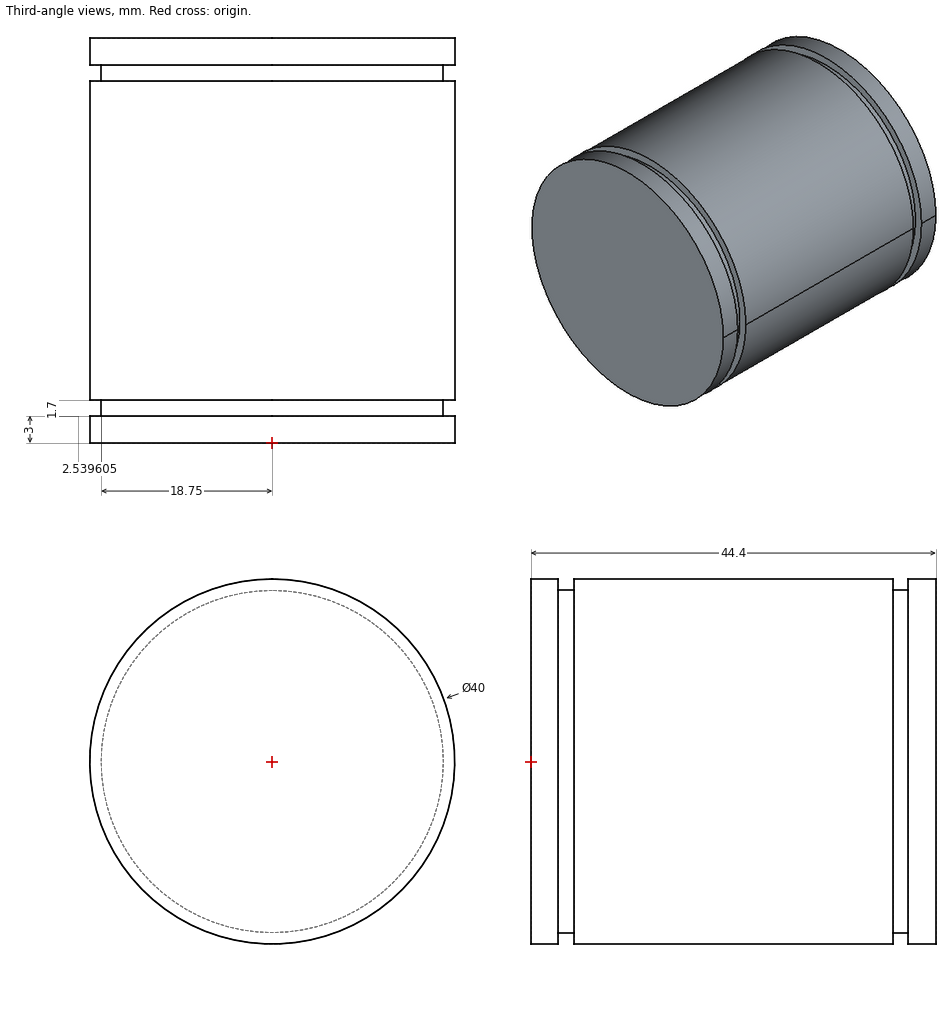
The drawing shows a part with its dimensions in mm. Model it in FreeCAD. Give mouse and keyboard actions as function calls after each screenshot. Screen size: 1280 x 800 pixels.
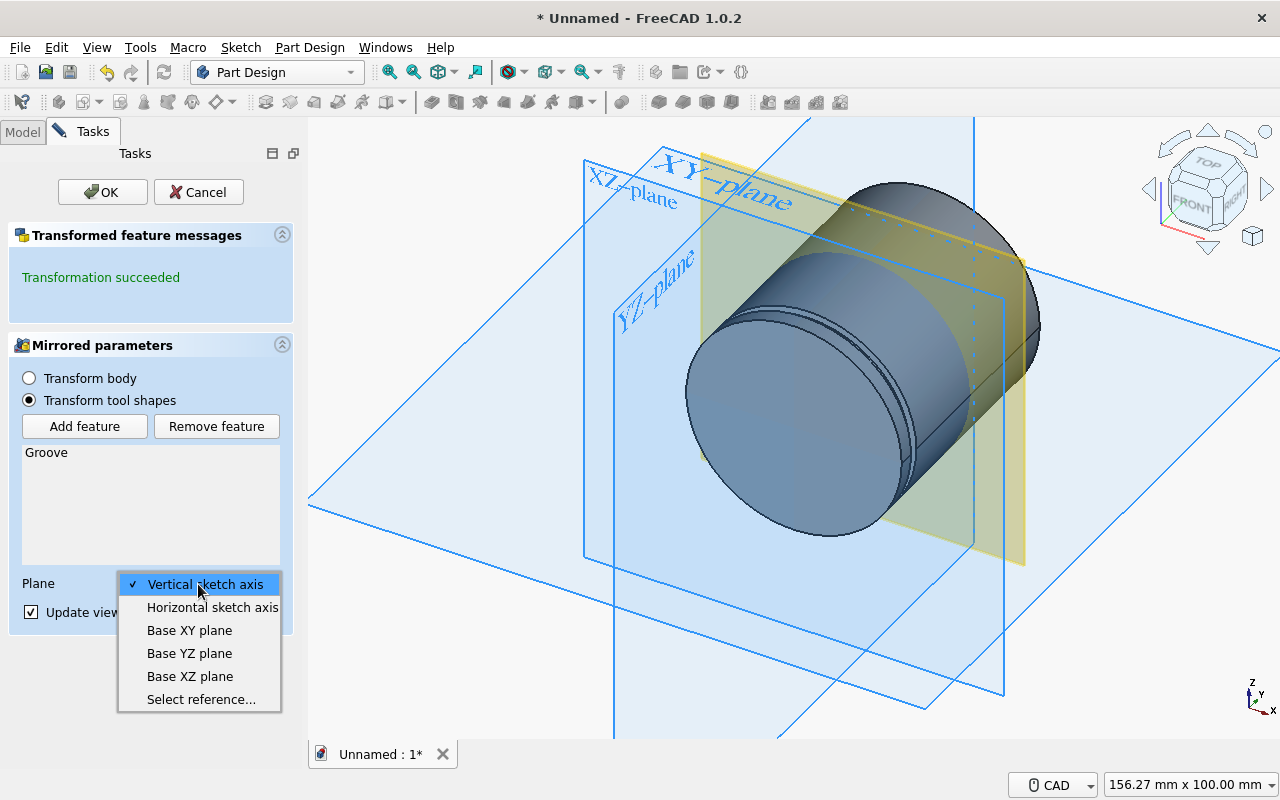
click(198, 700)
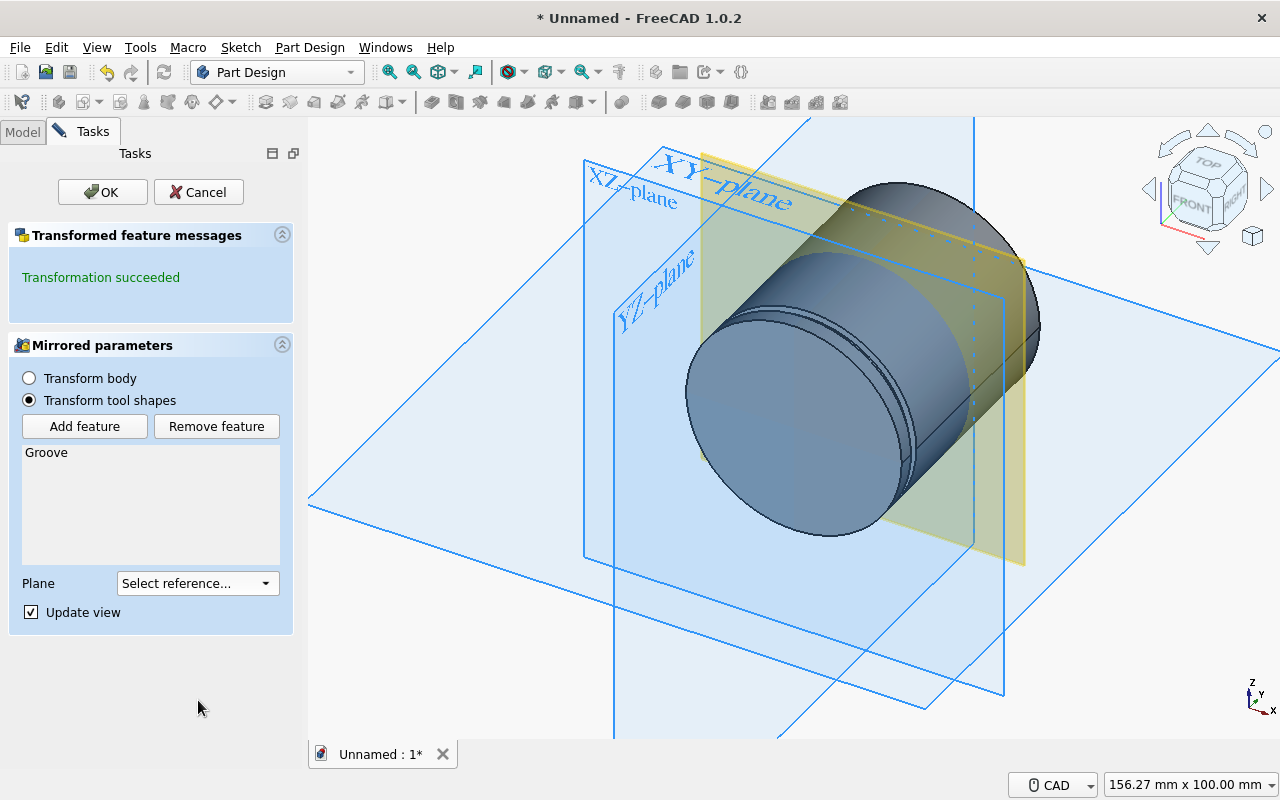
click(23, 131)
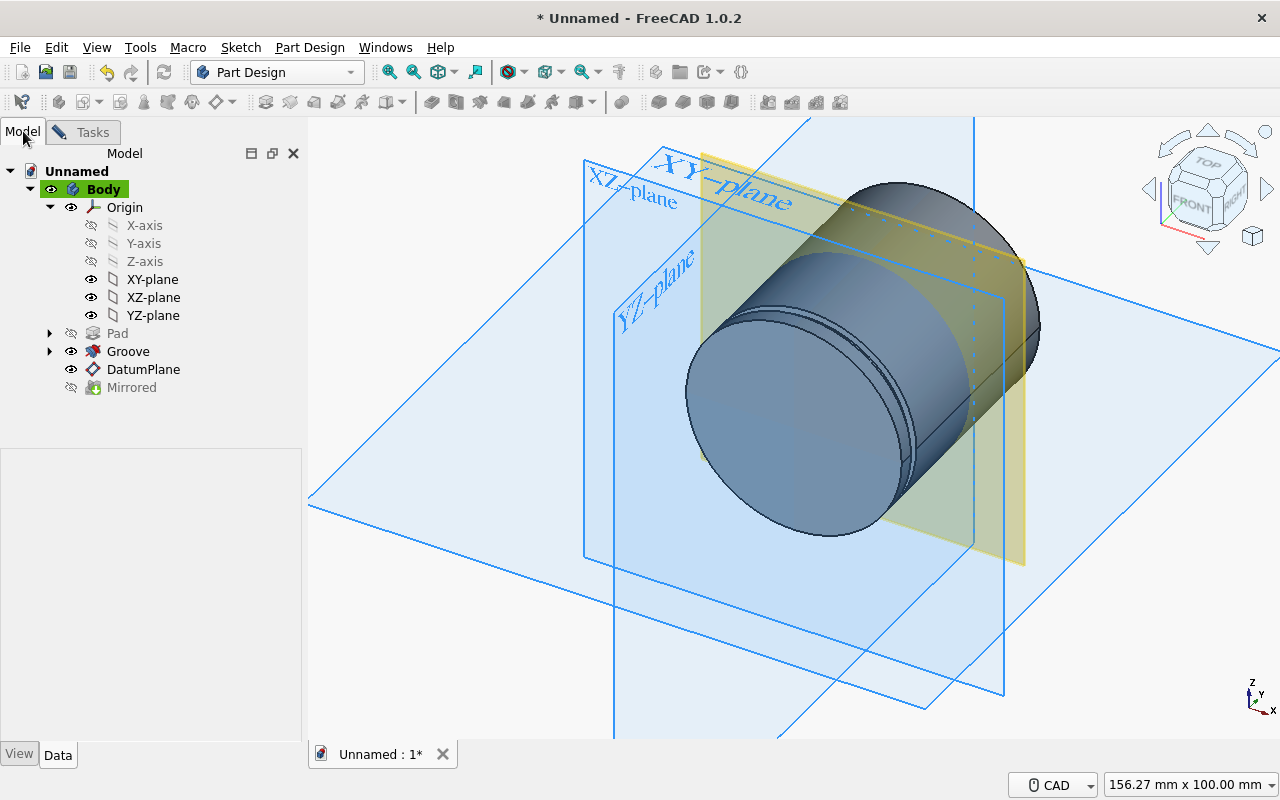
click(116, 369)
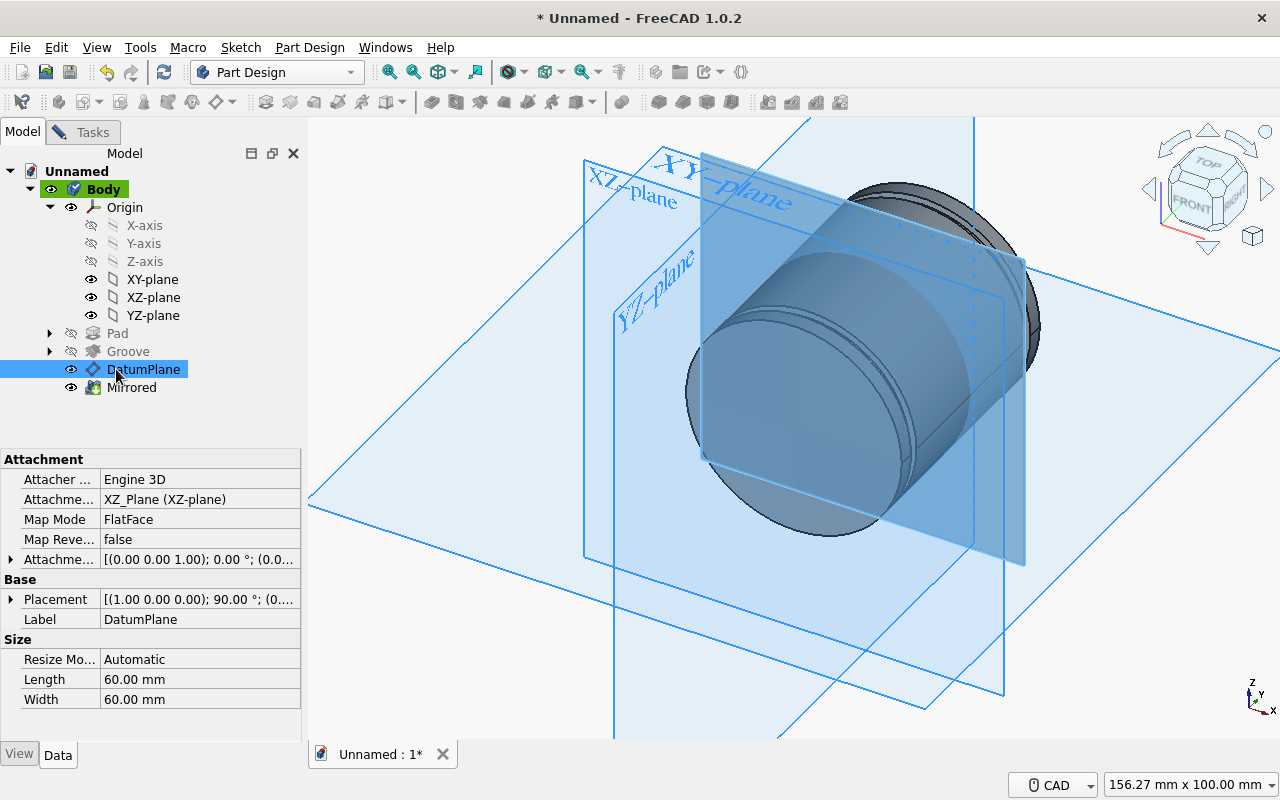
click(84, 131)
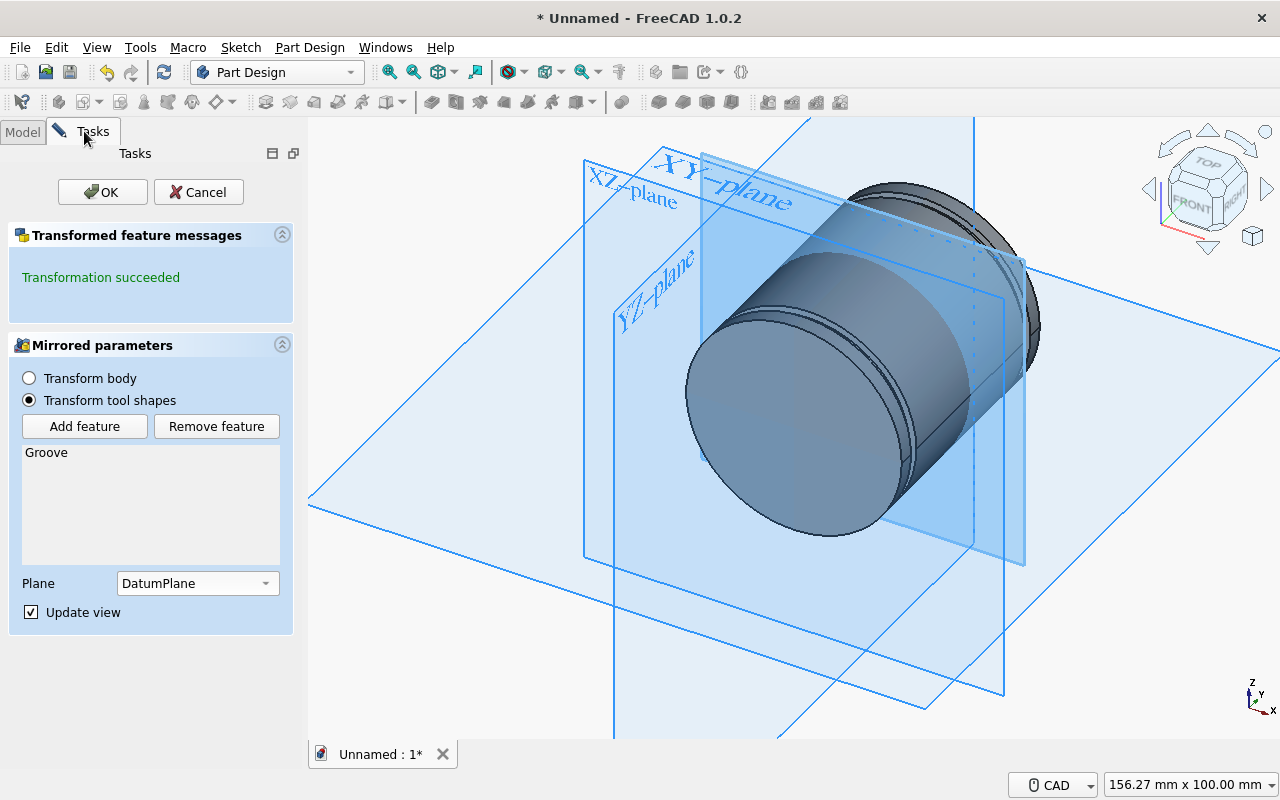
click(103, 192)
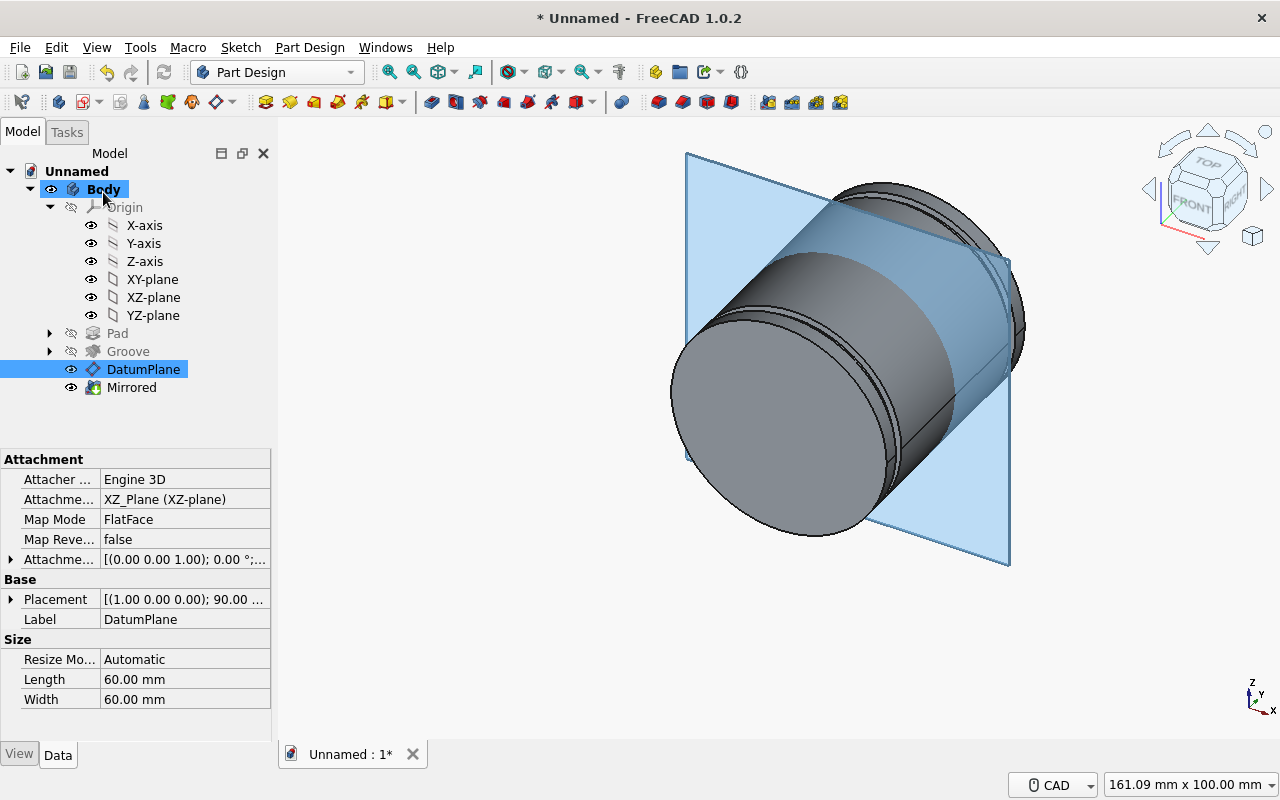
click(116, 369)
key(space)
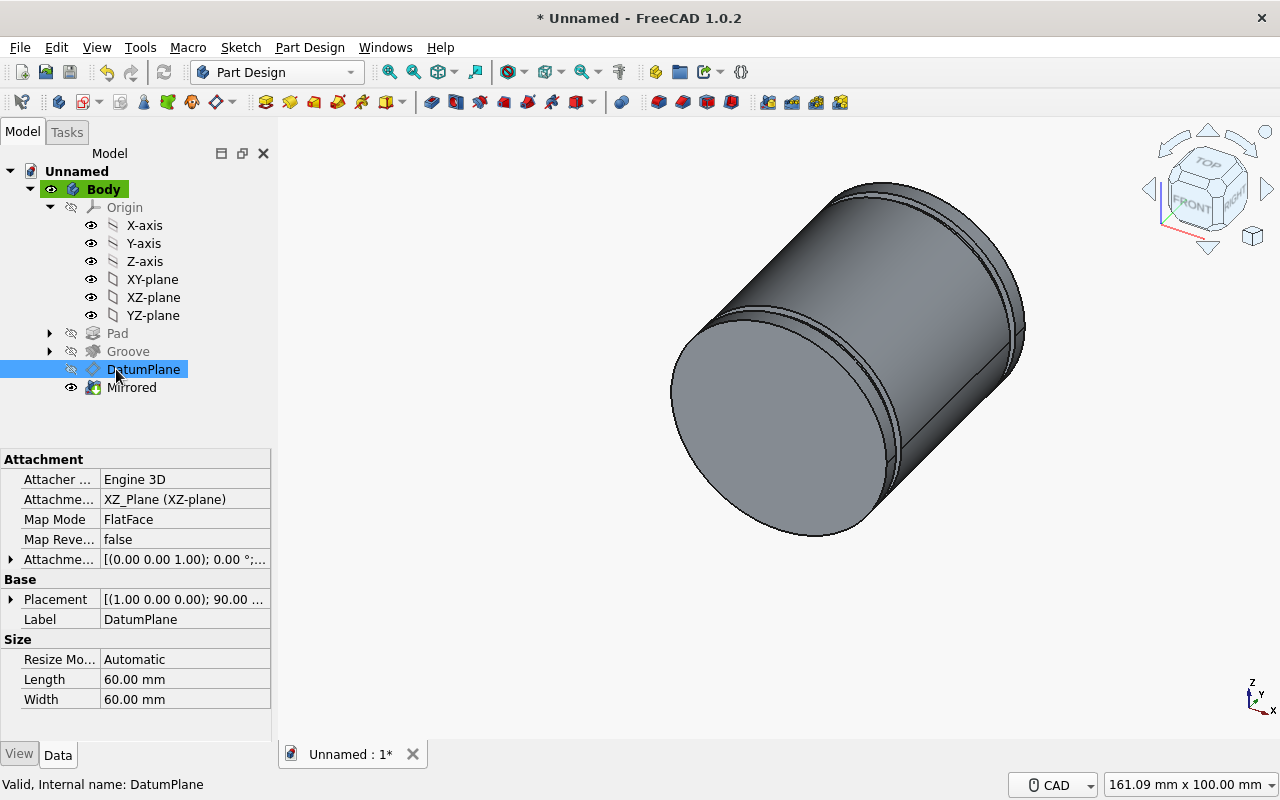
key(0)